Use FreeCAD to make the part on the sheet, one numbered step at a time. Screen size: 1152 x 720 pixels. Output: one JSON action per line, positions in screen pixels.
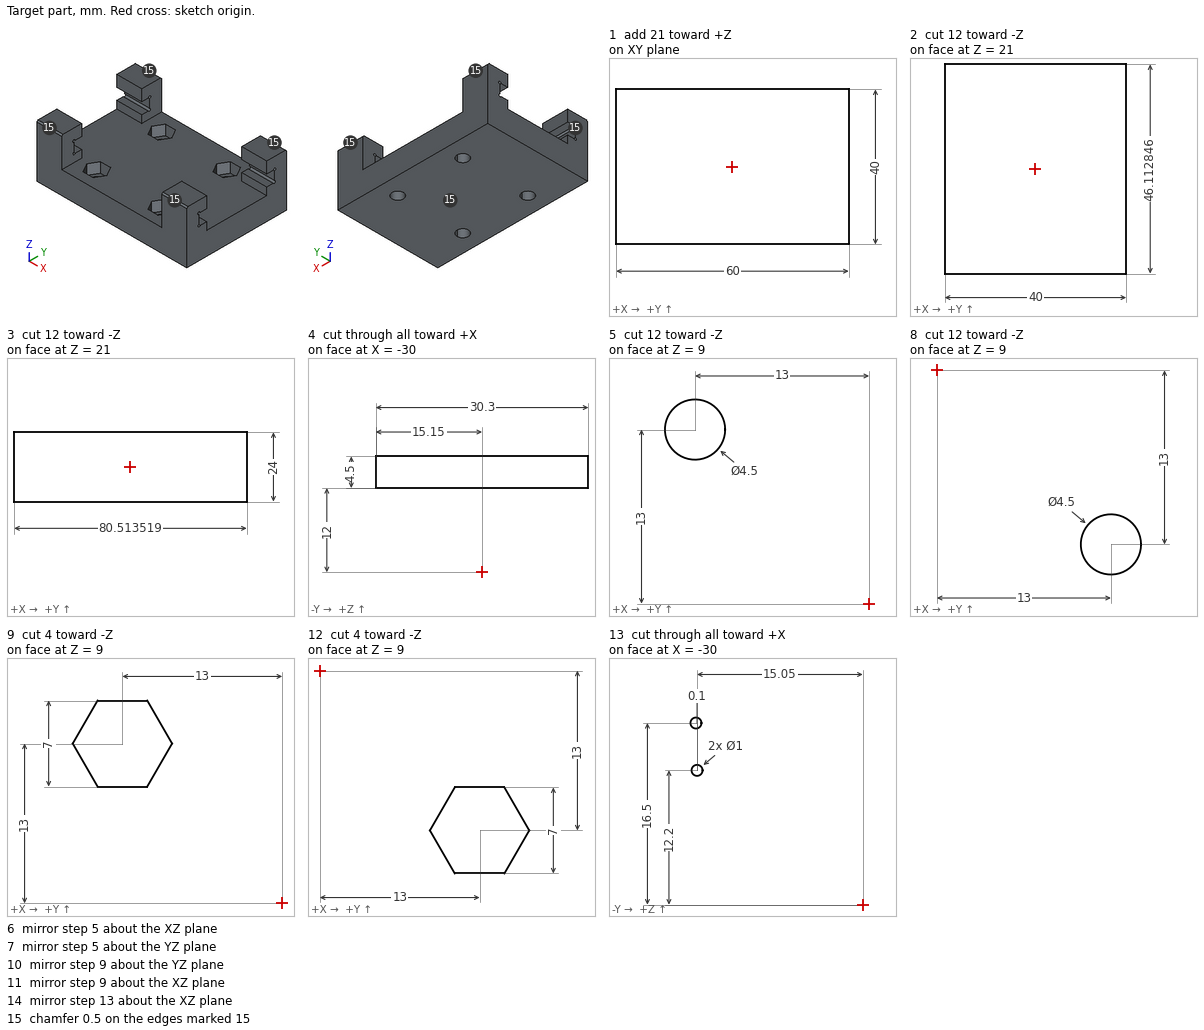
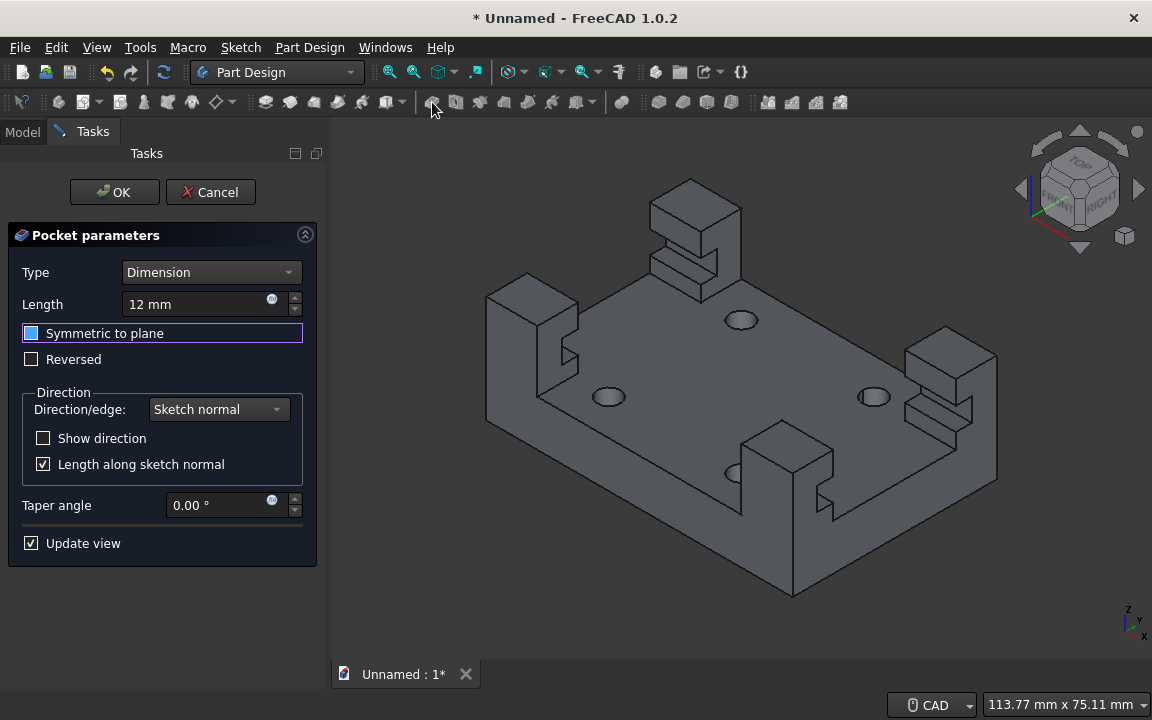
{"action": "left_click", "coordinate": [115, 192]}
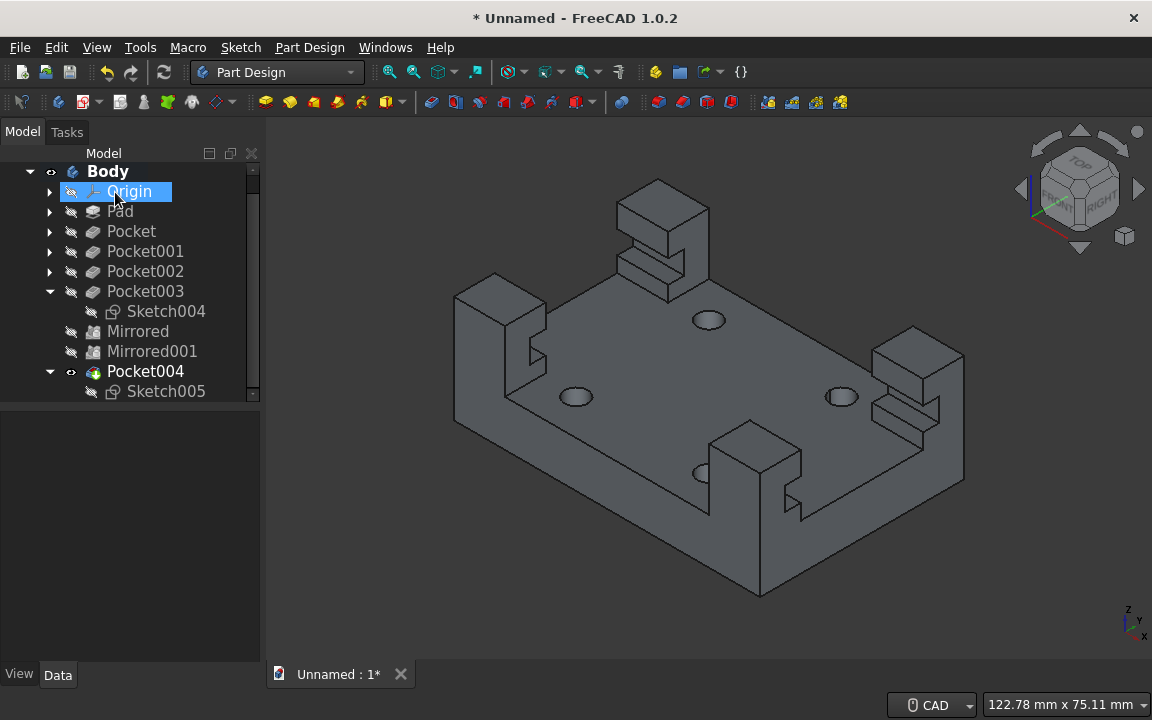
{"action": "left_click", "coordinate": [709, 396]}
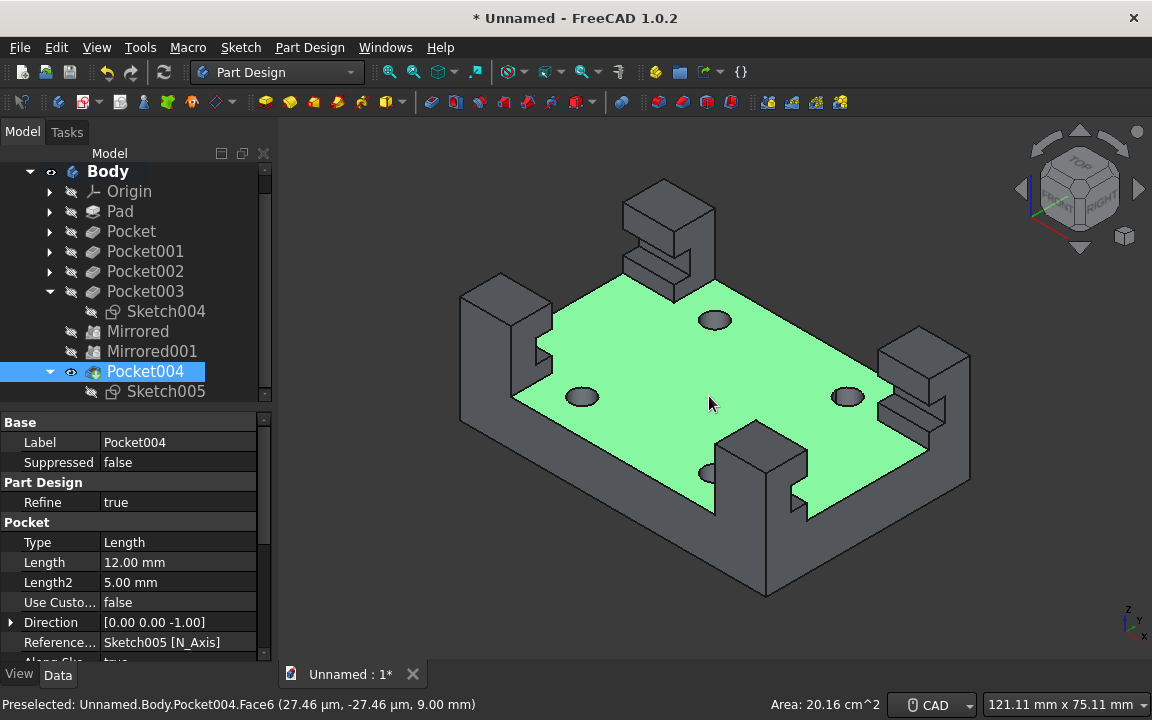
{"action": "left_click", "coordinate": [84, 102]}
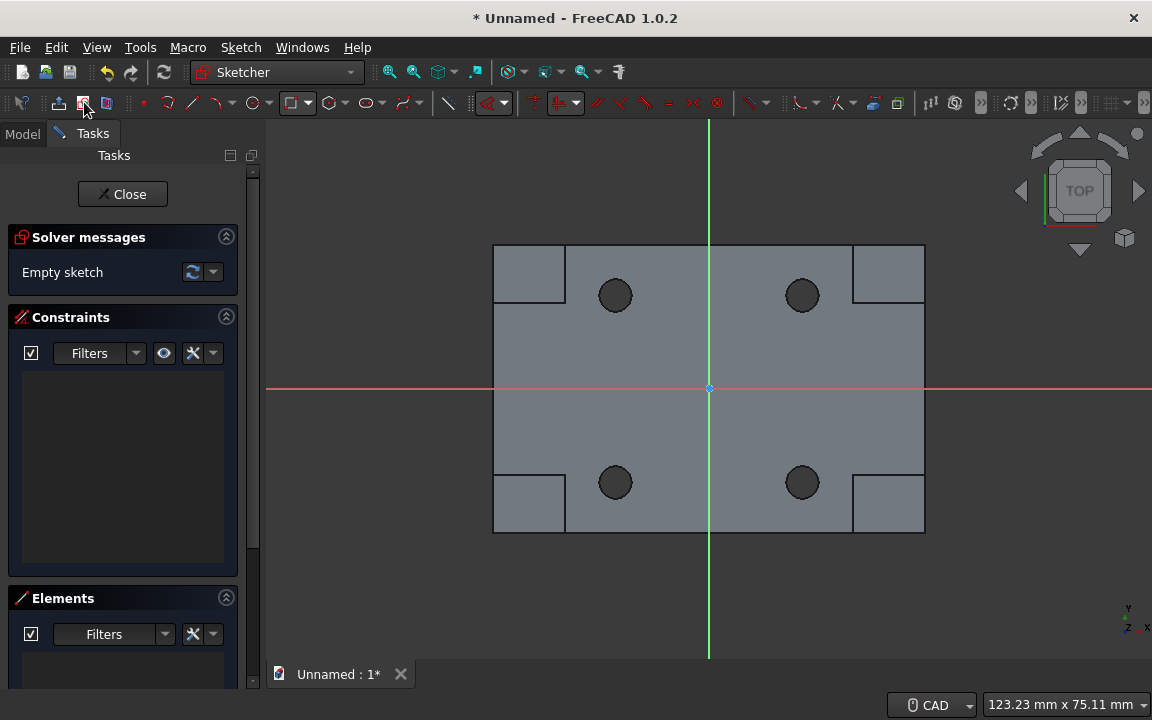
{"action": "left_click", "coordinate": [108, 104]}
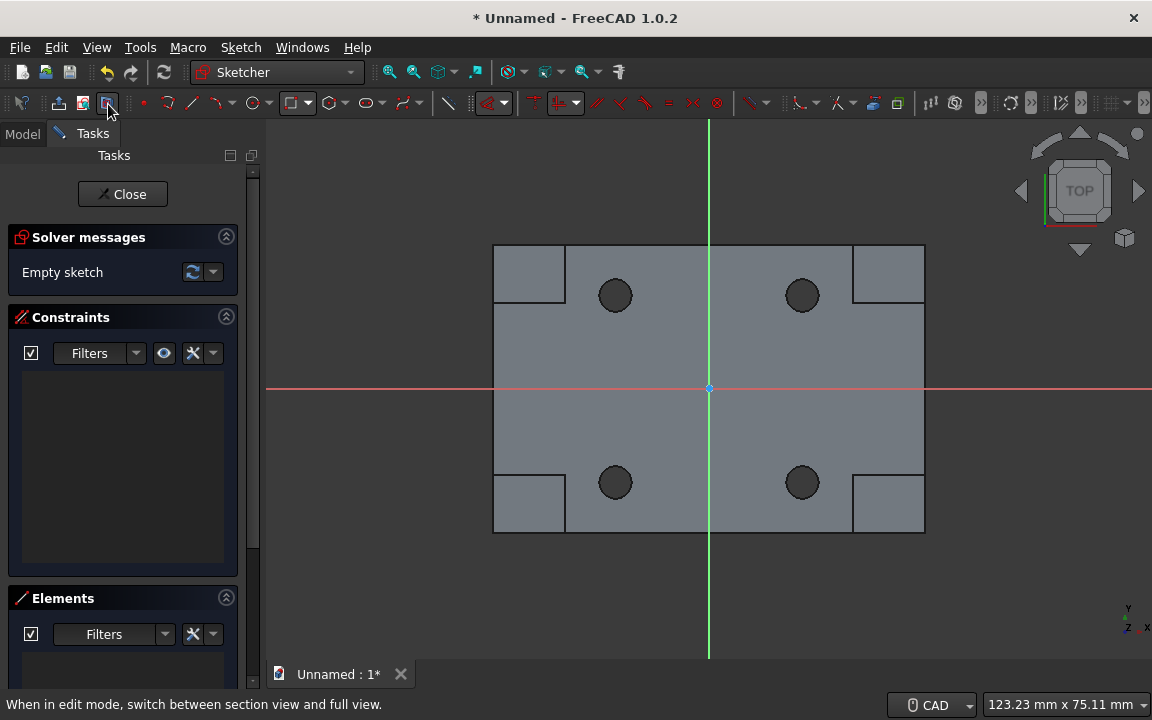
{"action": "scroll", "coordinate": [652, 295], "scroll_direction": "up", "scroll_amount": 5}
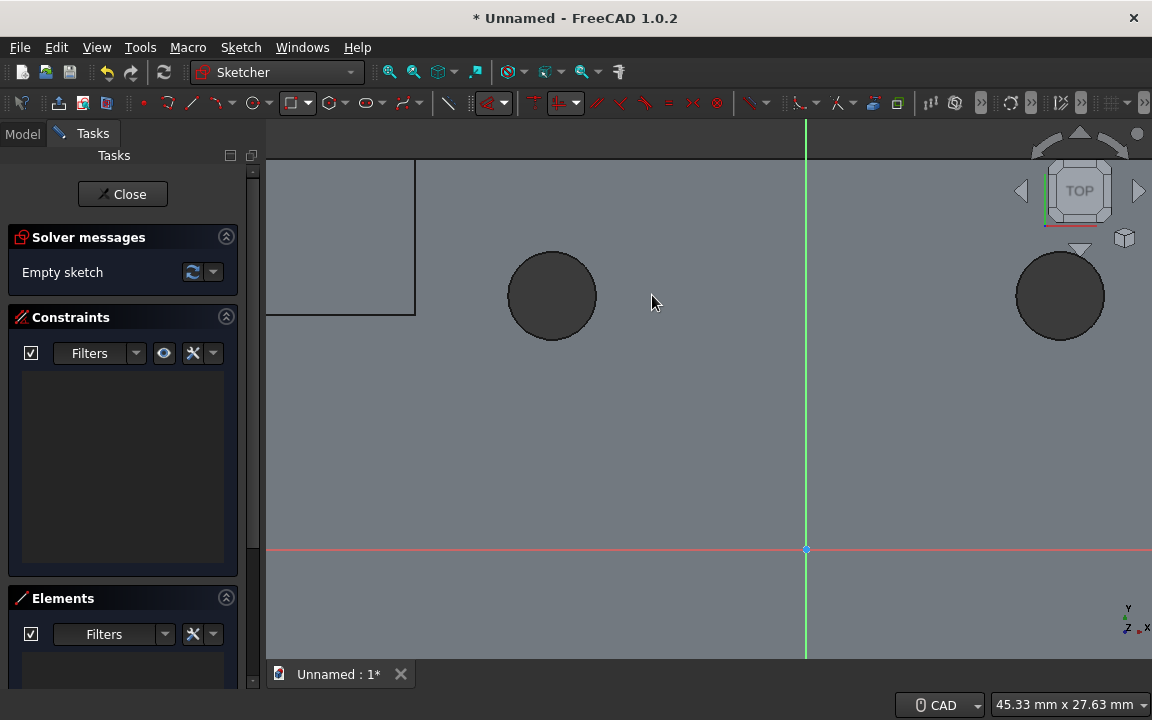
{"action": "left_click", "coordinate": [330, 104]}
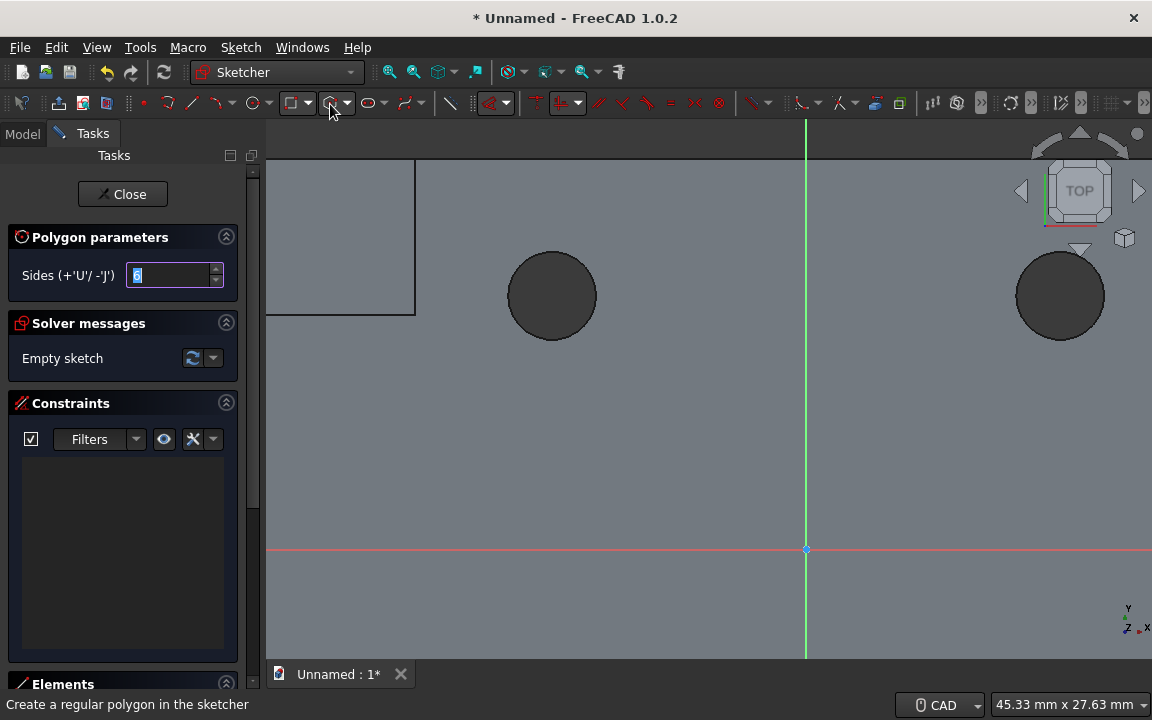
{"action": "left_click", "coordinate": [552, 296]}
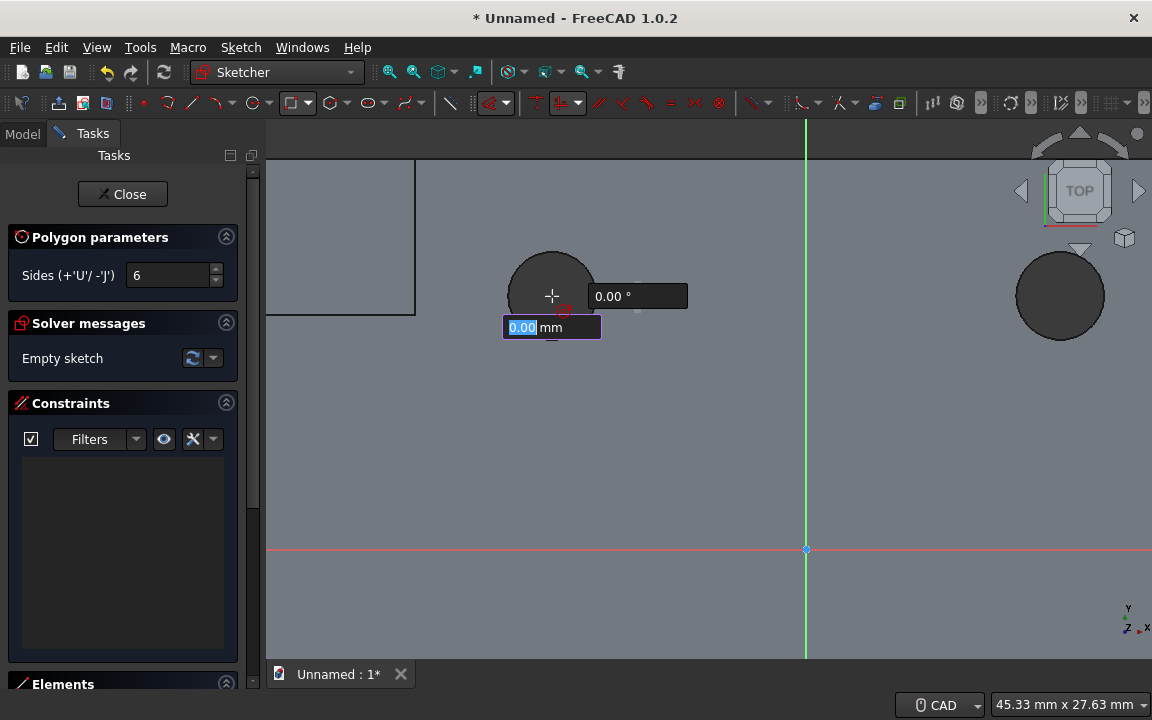
{"action": "left_click", "coordinate": [473, 296]}
{"action": "key", "text": "Escape"}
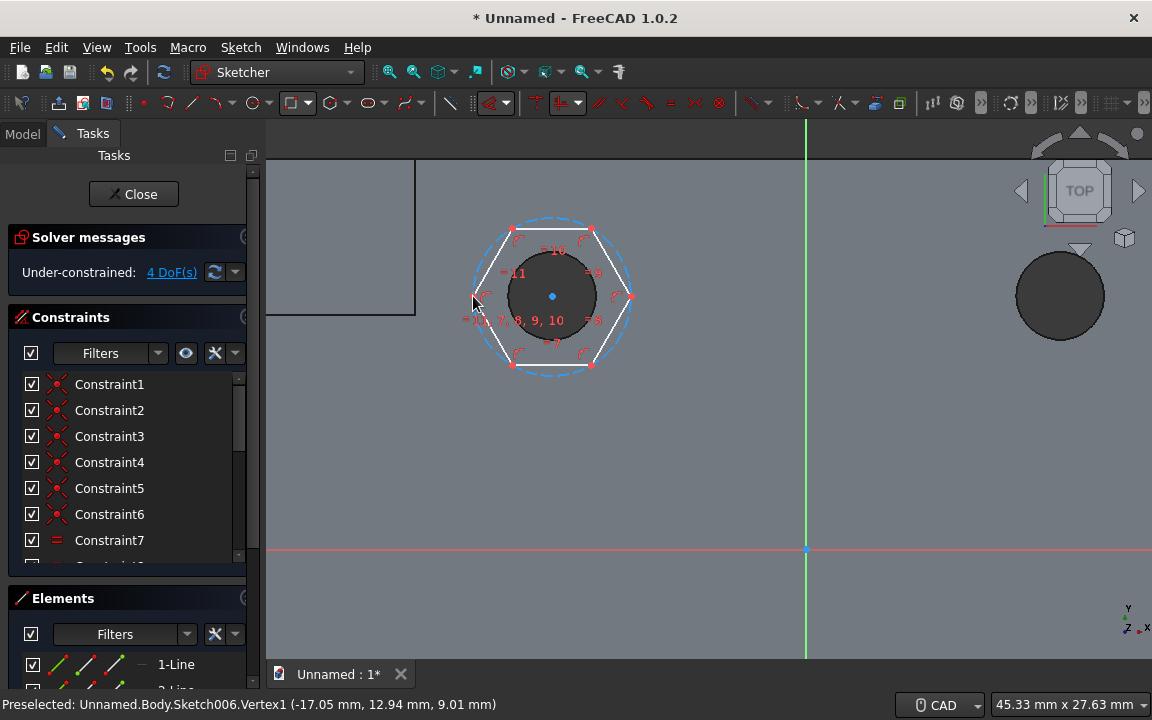
{"action": "scroll", "coordinate": [544, 365], "scroll_direction": "up", "scroll_amount": 2}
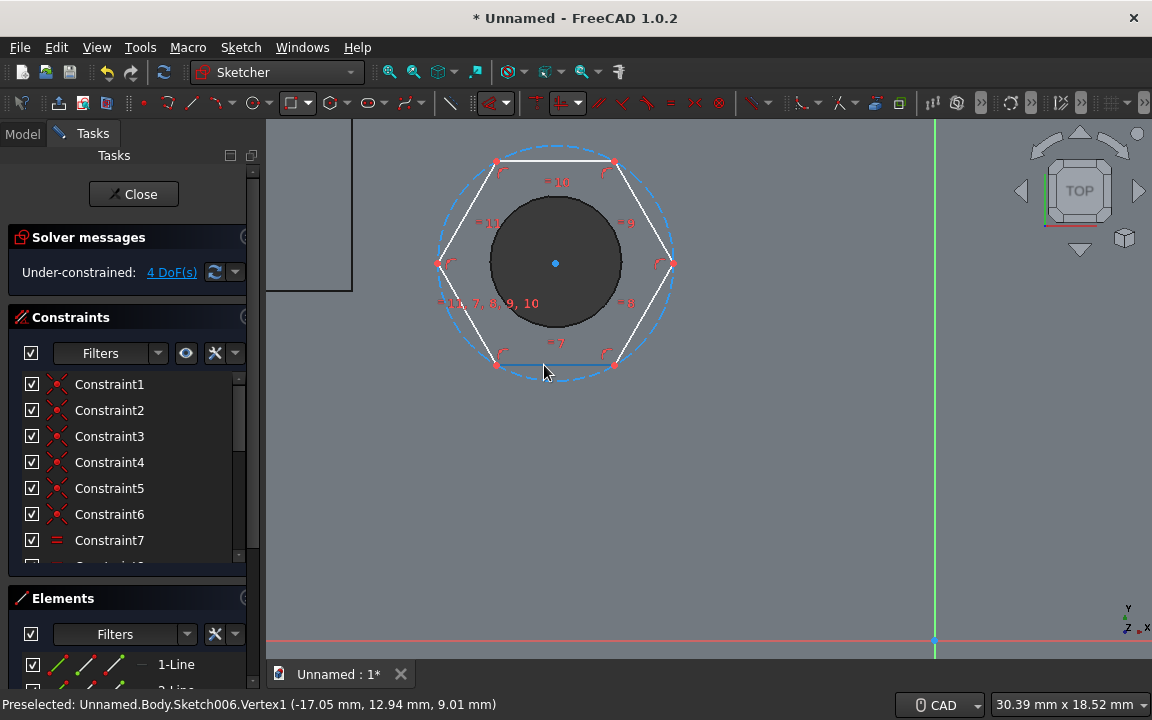
{"action": "left_click", "coordinate": [544, 365]}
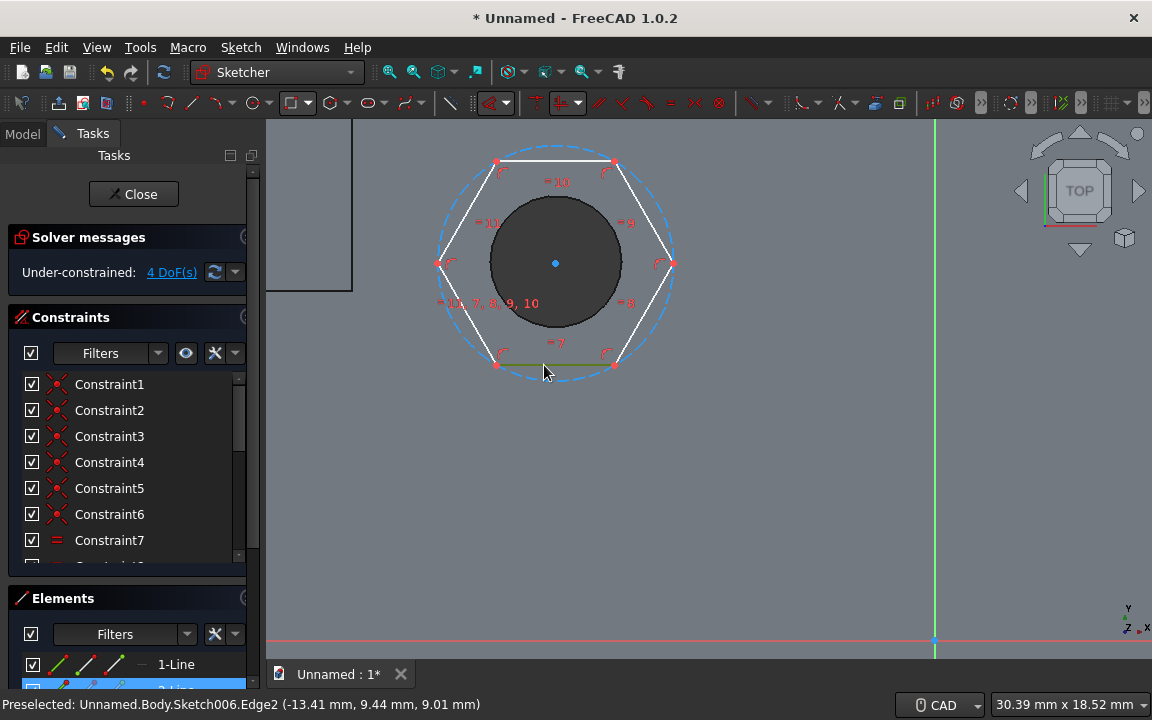
{"action": "key", "text": "h"}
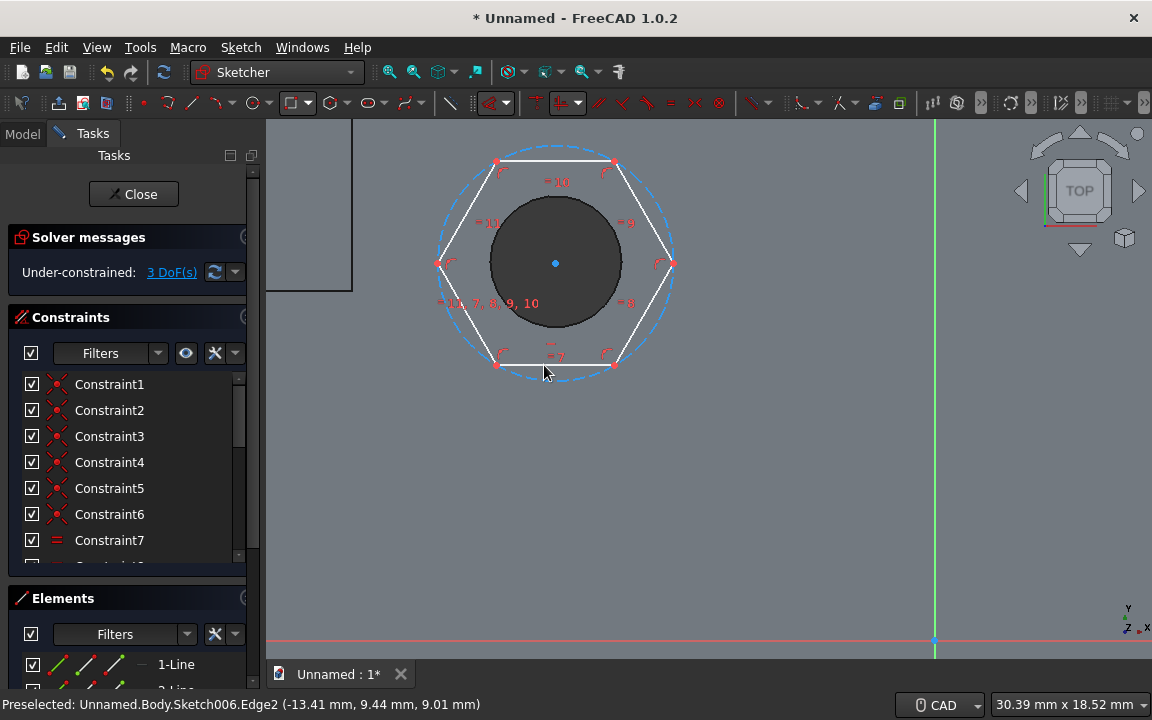
{"action": "left_click", "coordinate": [497, 365]}